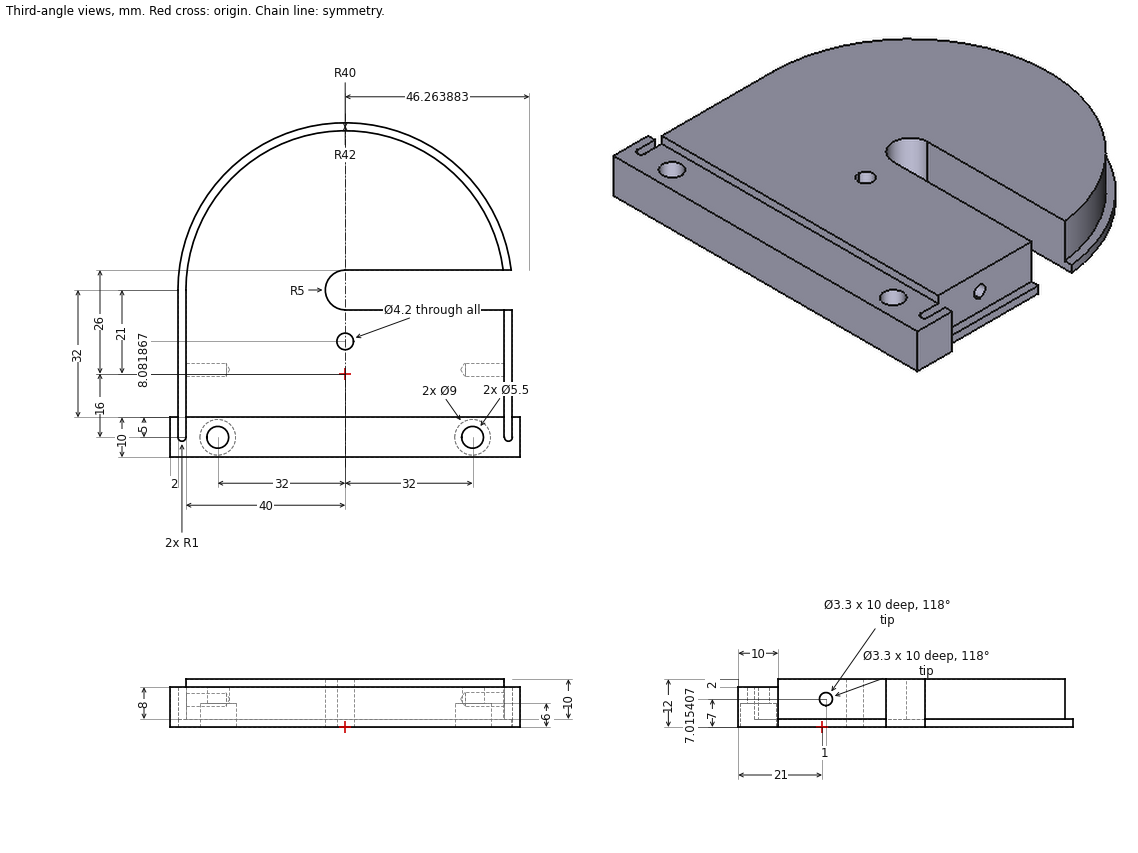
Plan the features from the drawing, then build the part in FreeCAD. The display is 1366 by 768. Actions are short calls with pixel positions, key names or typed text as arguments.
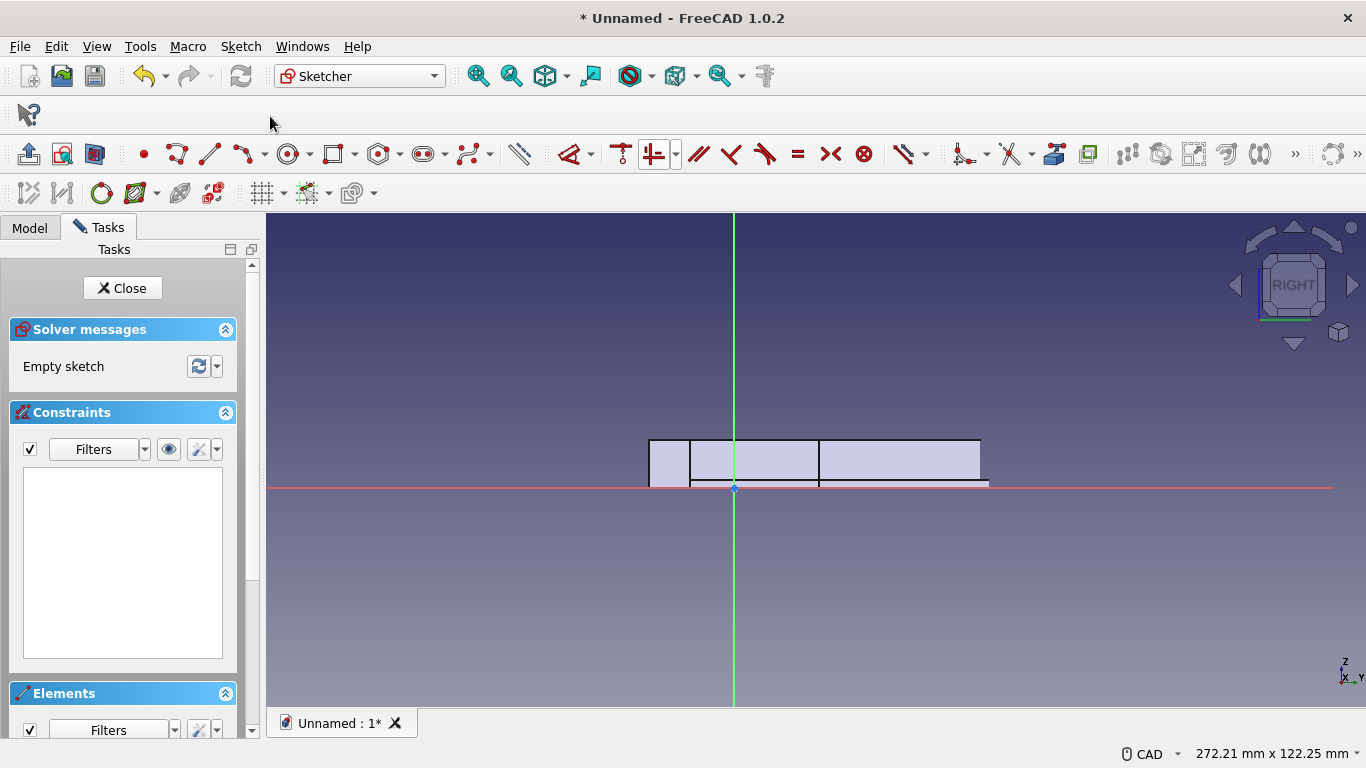
scroll(681, 465, up, 9)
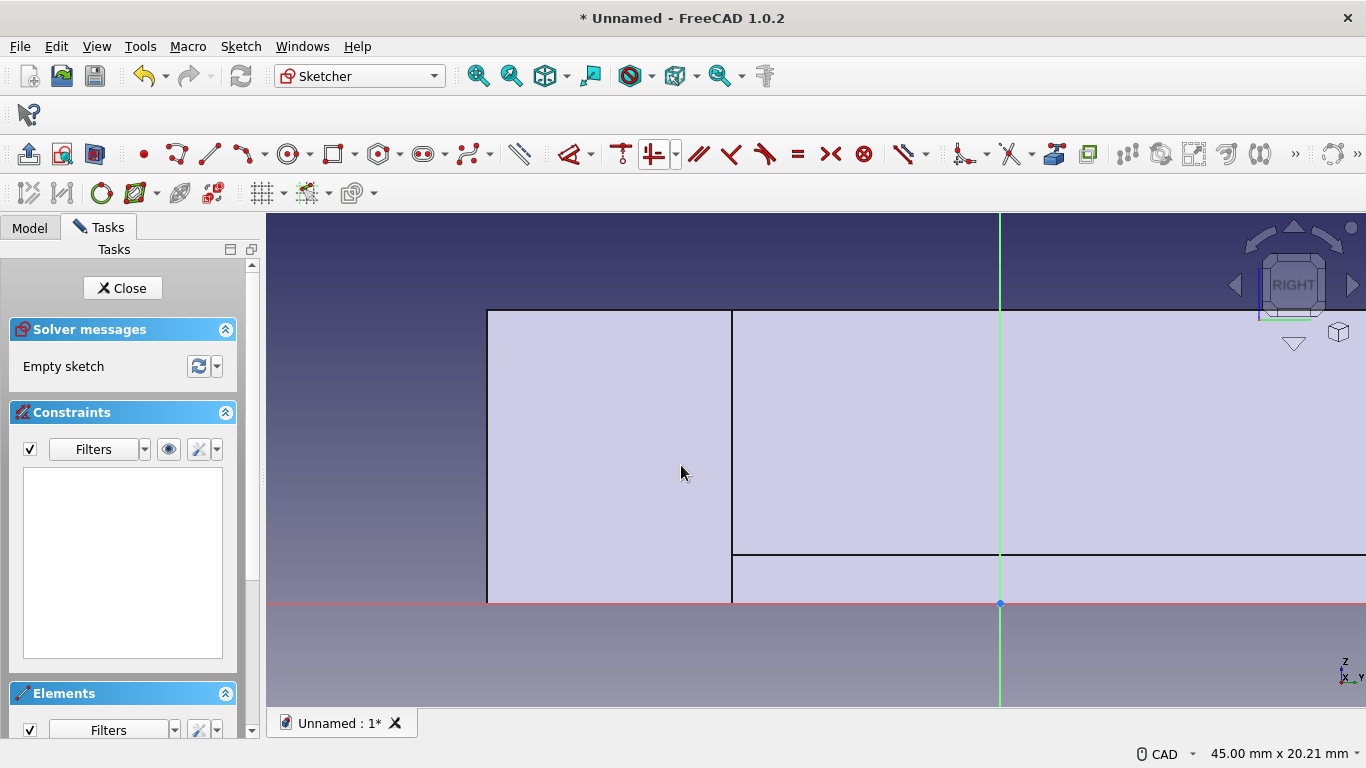
click(332, 154)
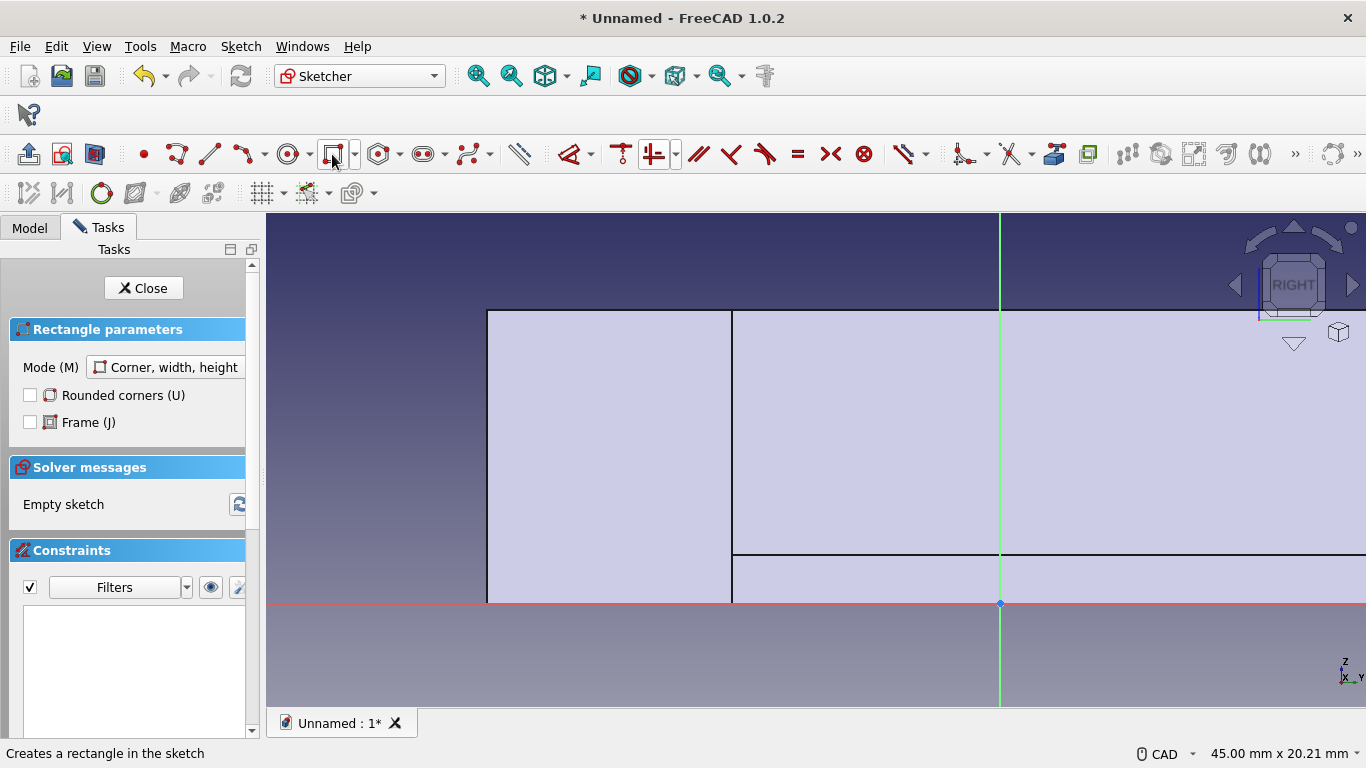
click(487, 310)
click(732, 359)
key(Escape)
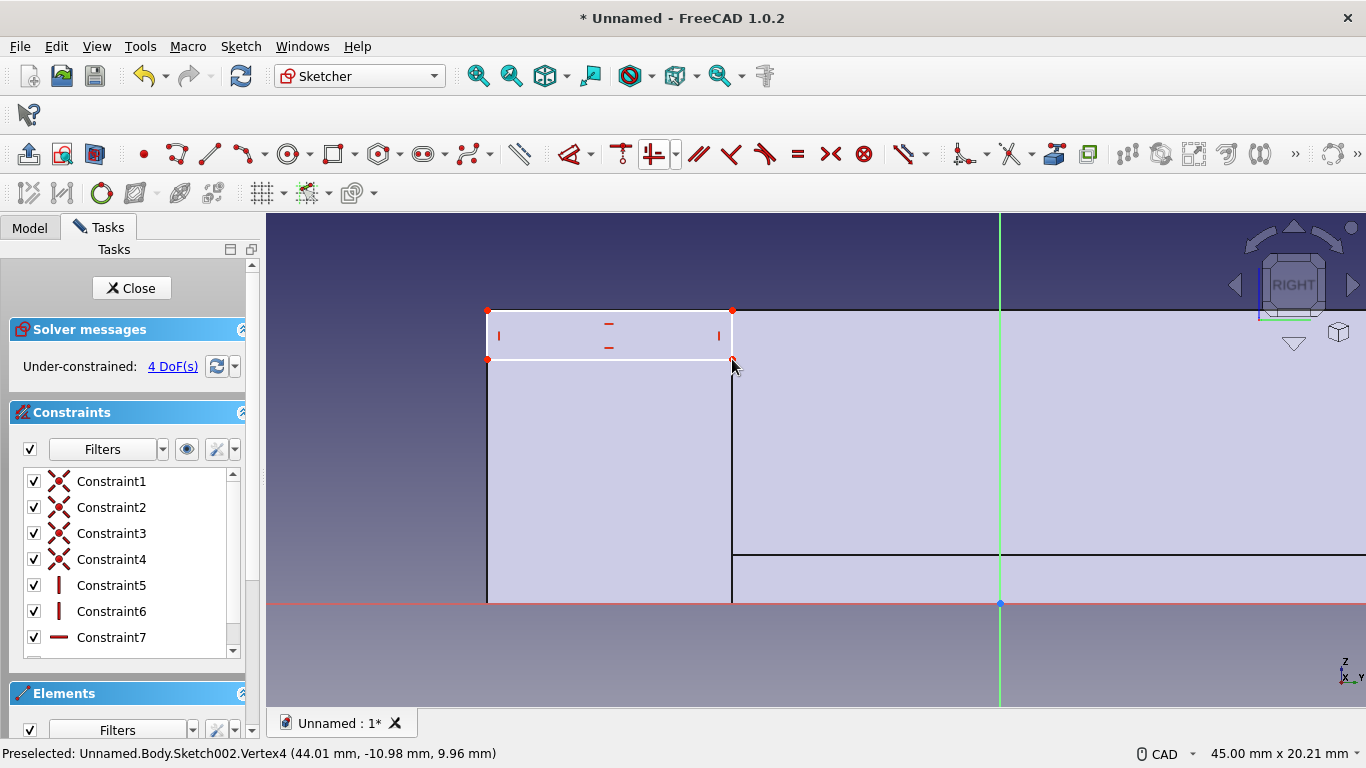
click(568, 154)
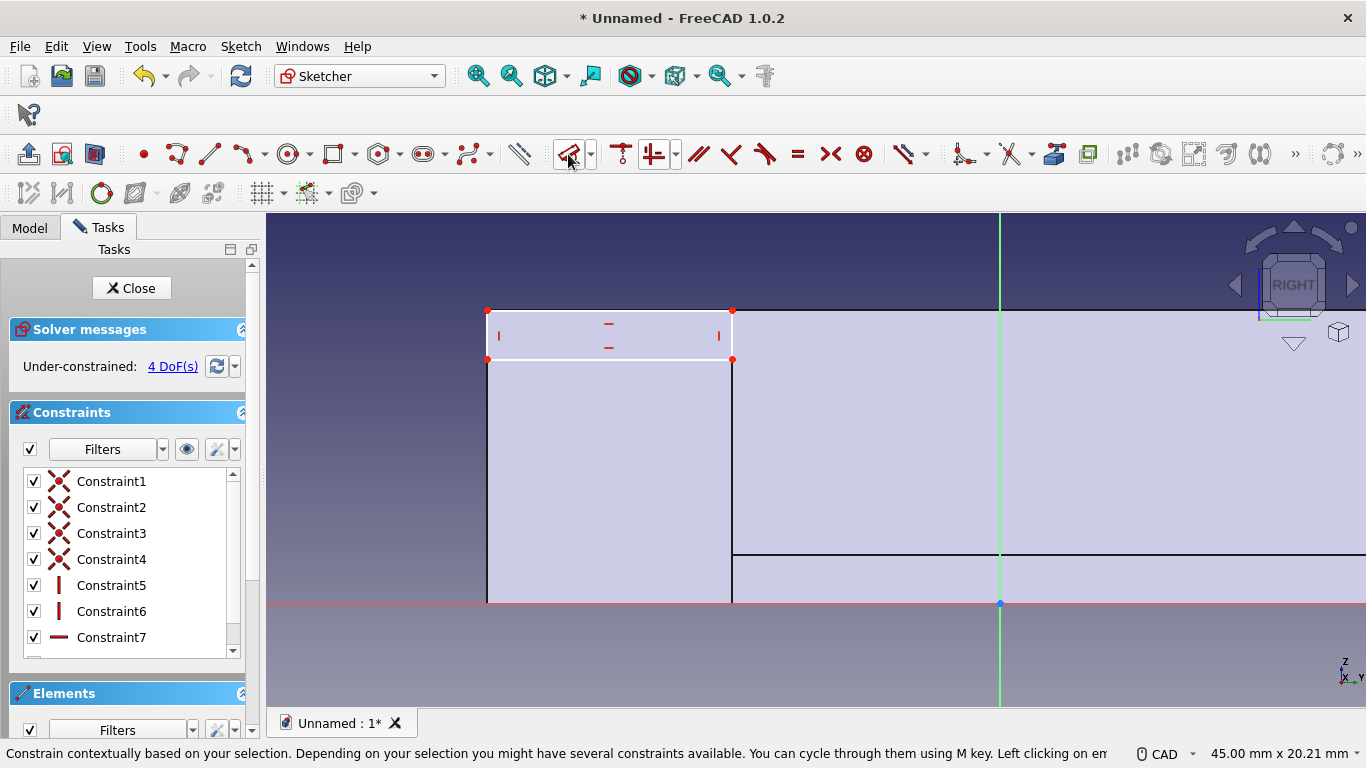
click(487, 326)
click(453, 336)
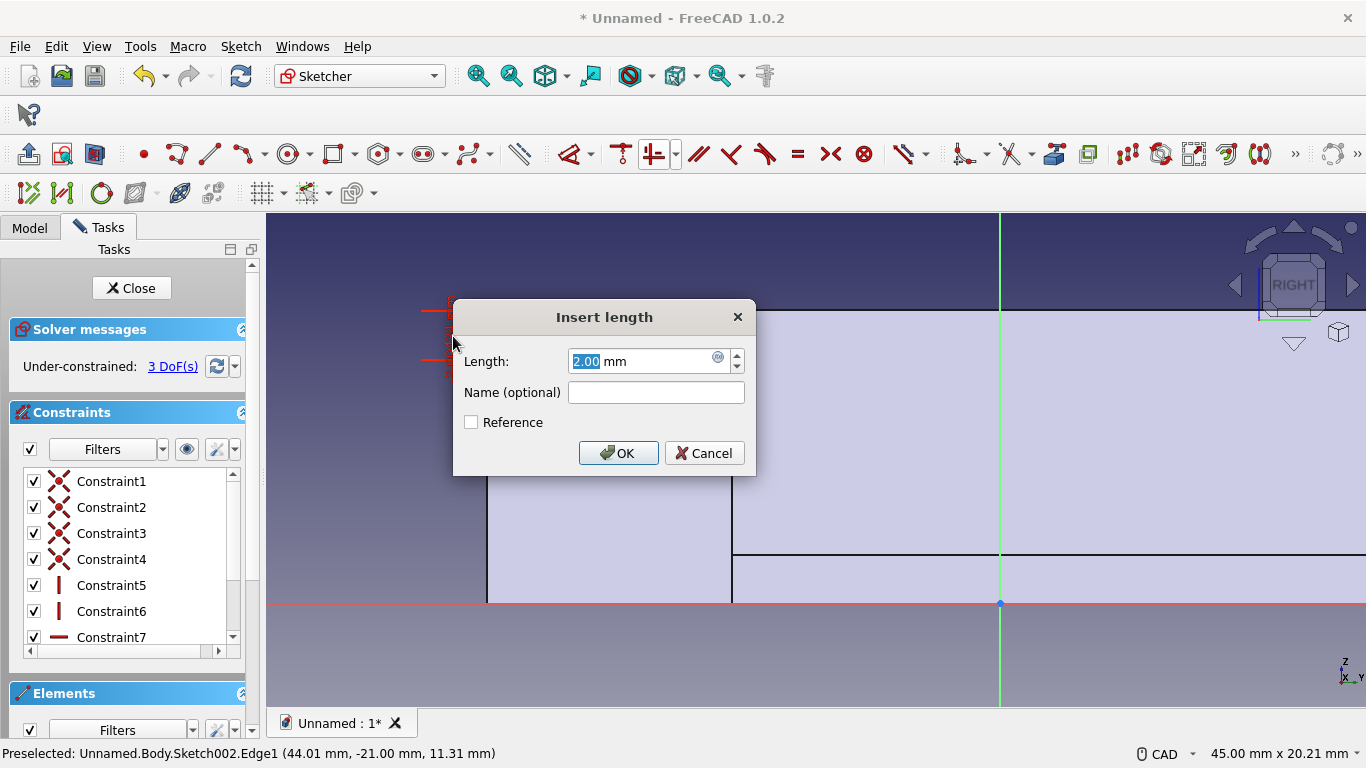
text(2)
key(Return)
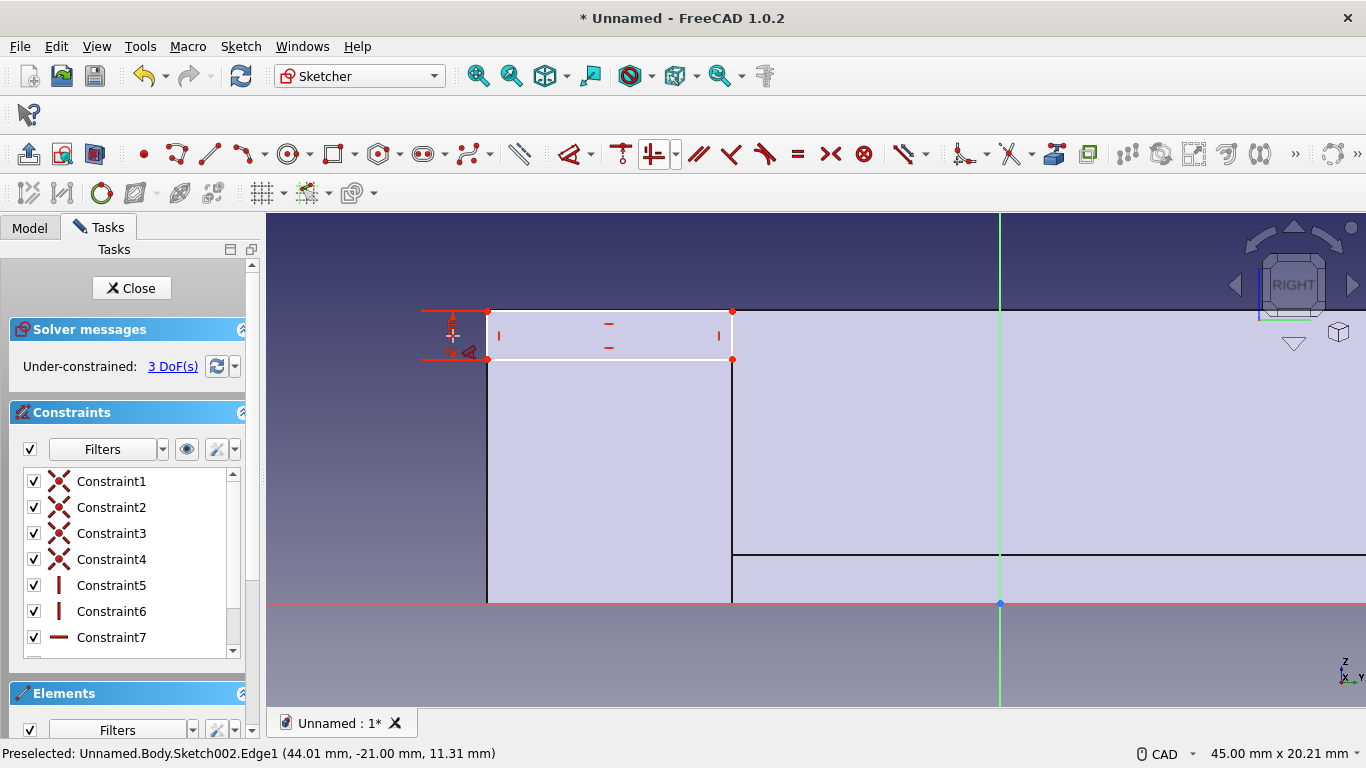
click(561, 360)
click(610, 326)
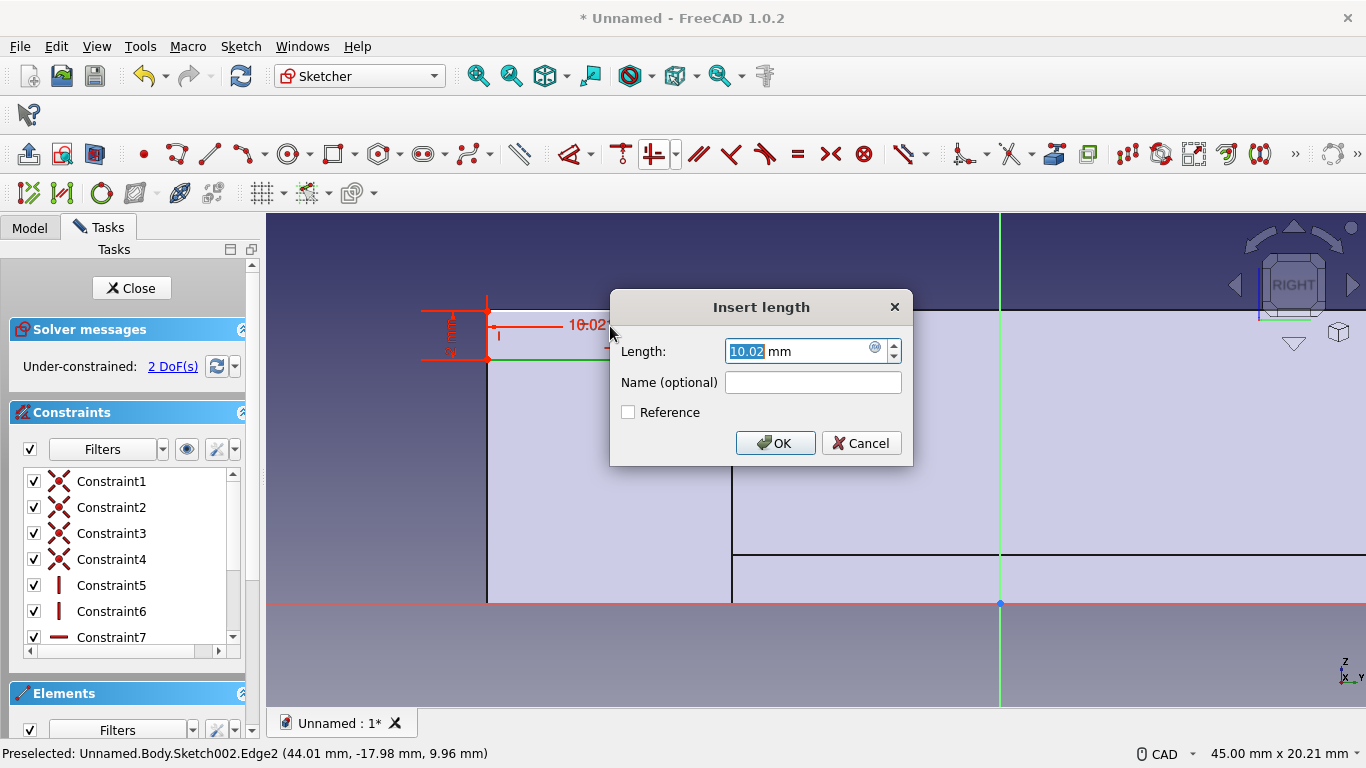
text(10)
key(Return)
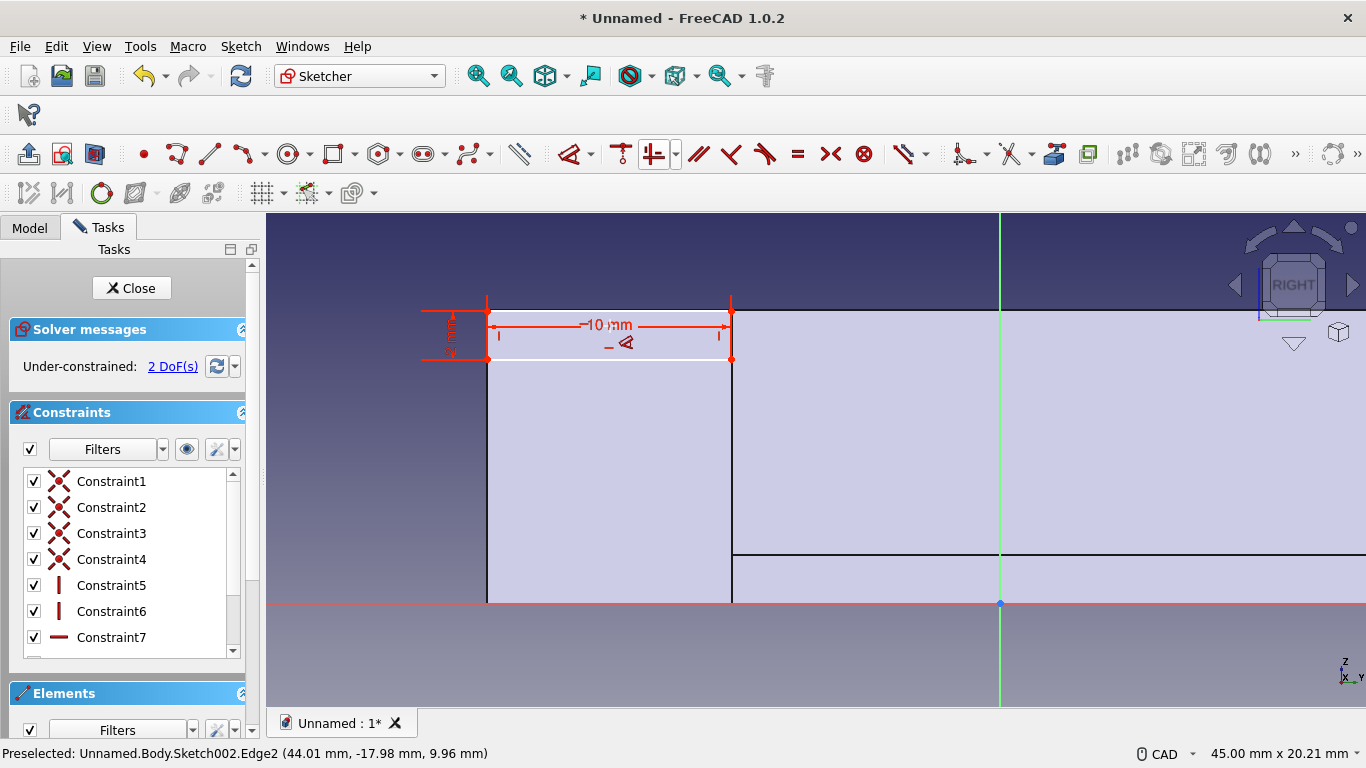
click(487, 311)
click(744, 638)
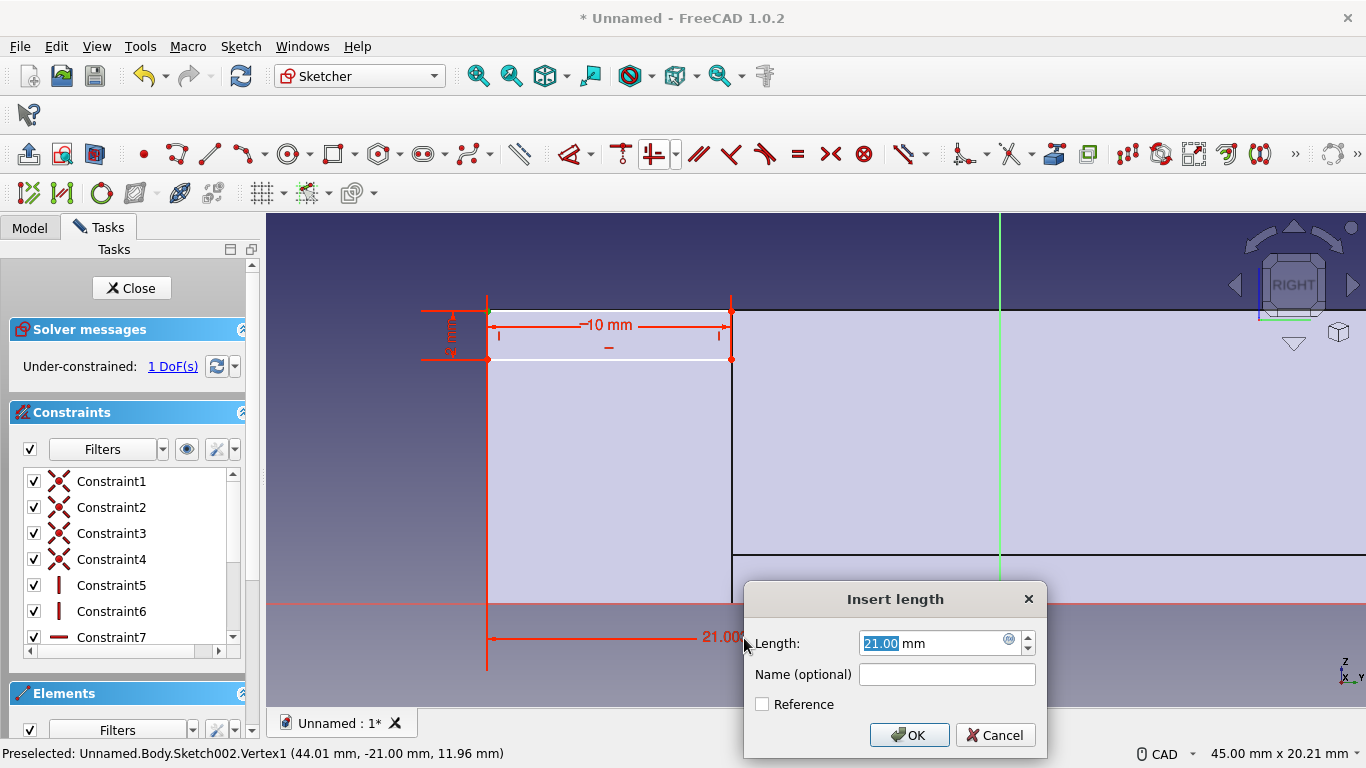
text(21)
key(Return)